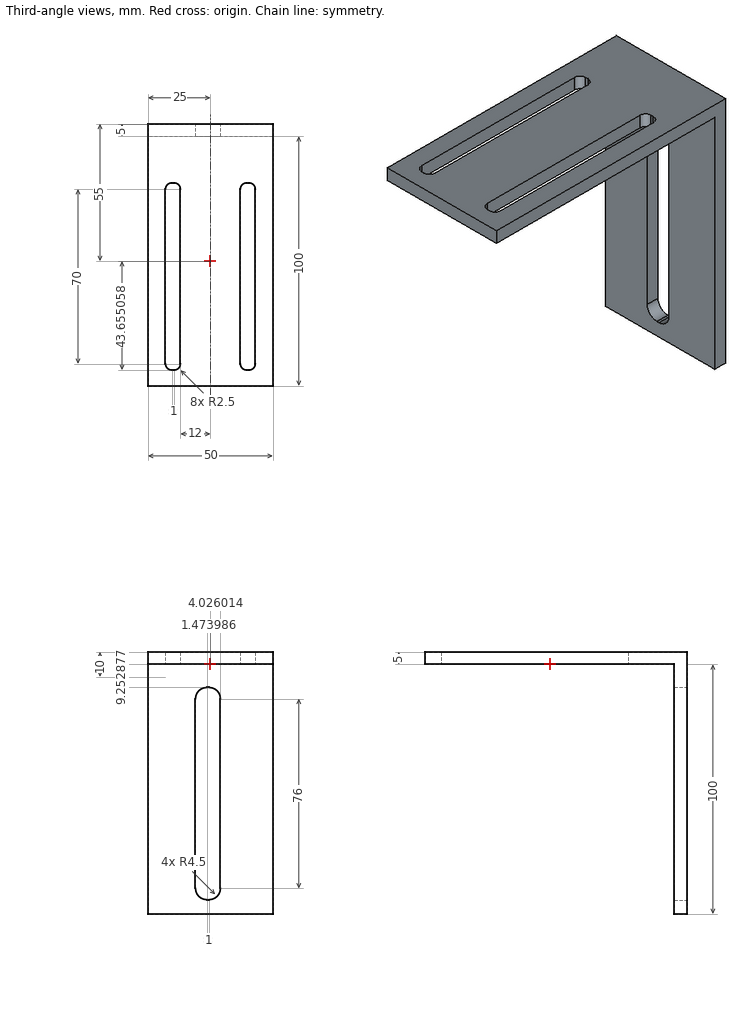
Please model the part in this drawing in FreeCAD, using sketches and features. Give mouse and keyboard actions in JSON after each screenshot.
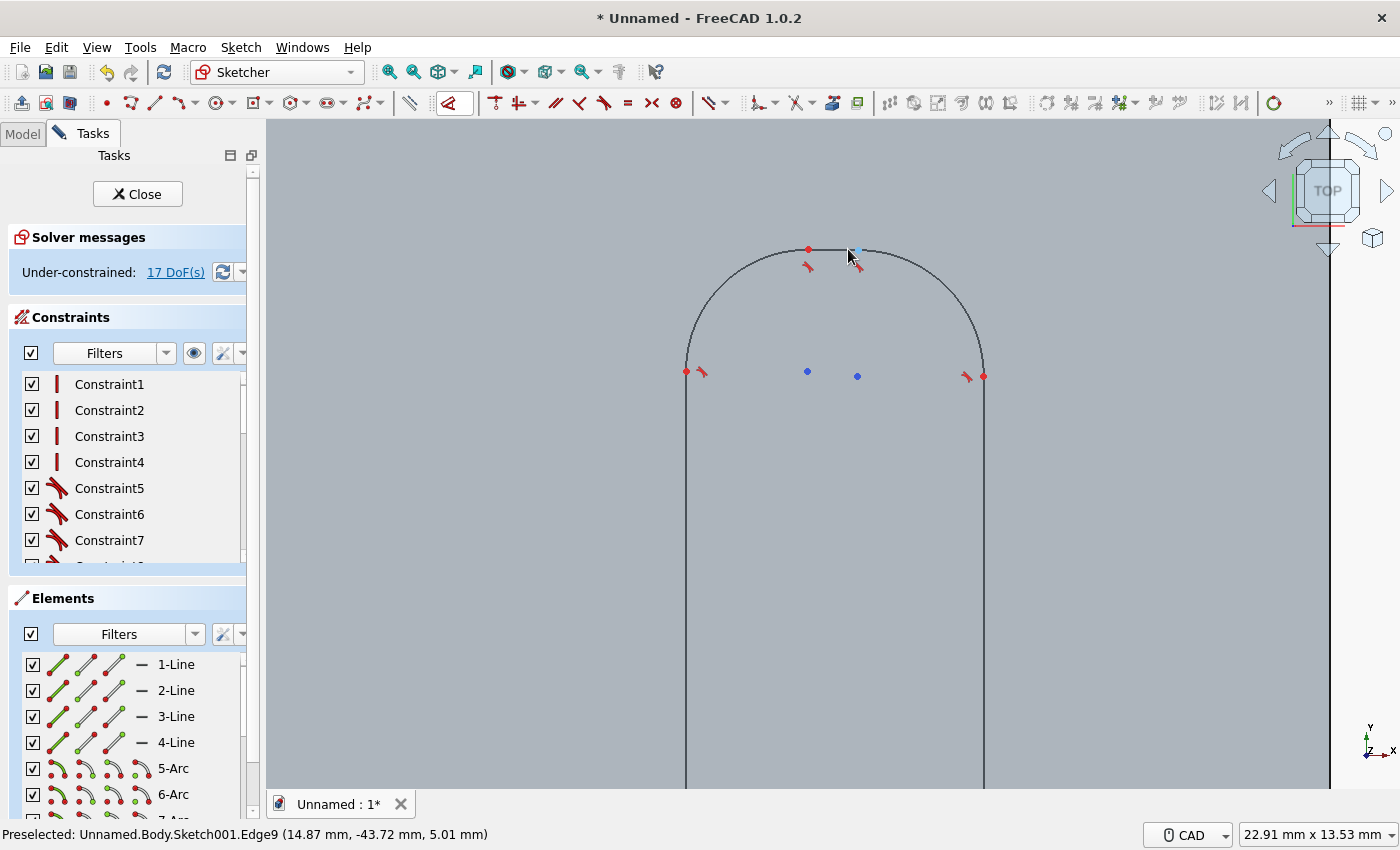
{"action": "left_click", "coordinate": [843, 250]}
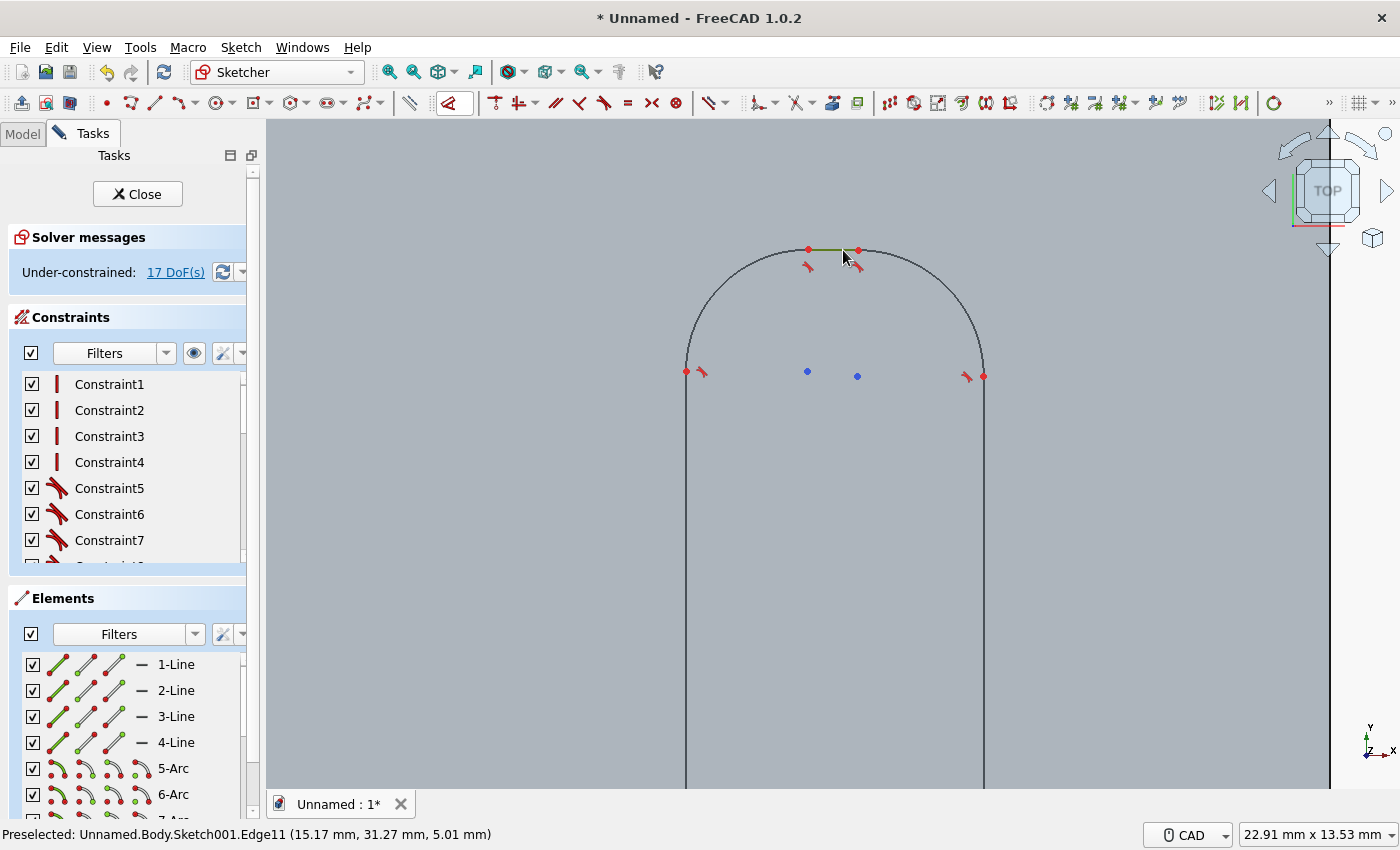
{"action": "key", "text": "h"}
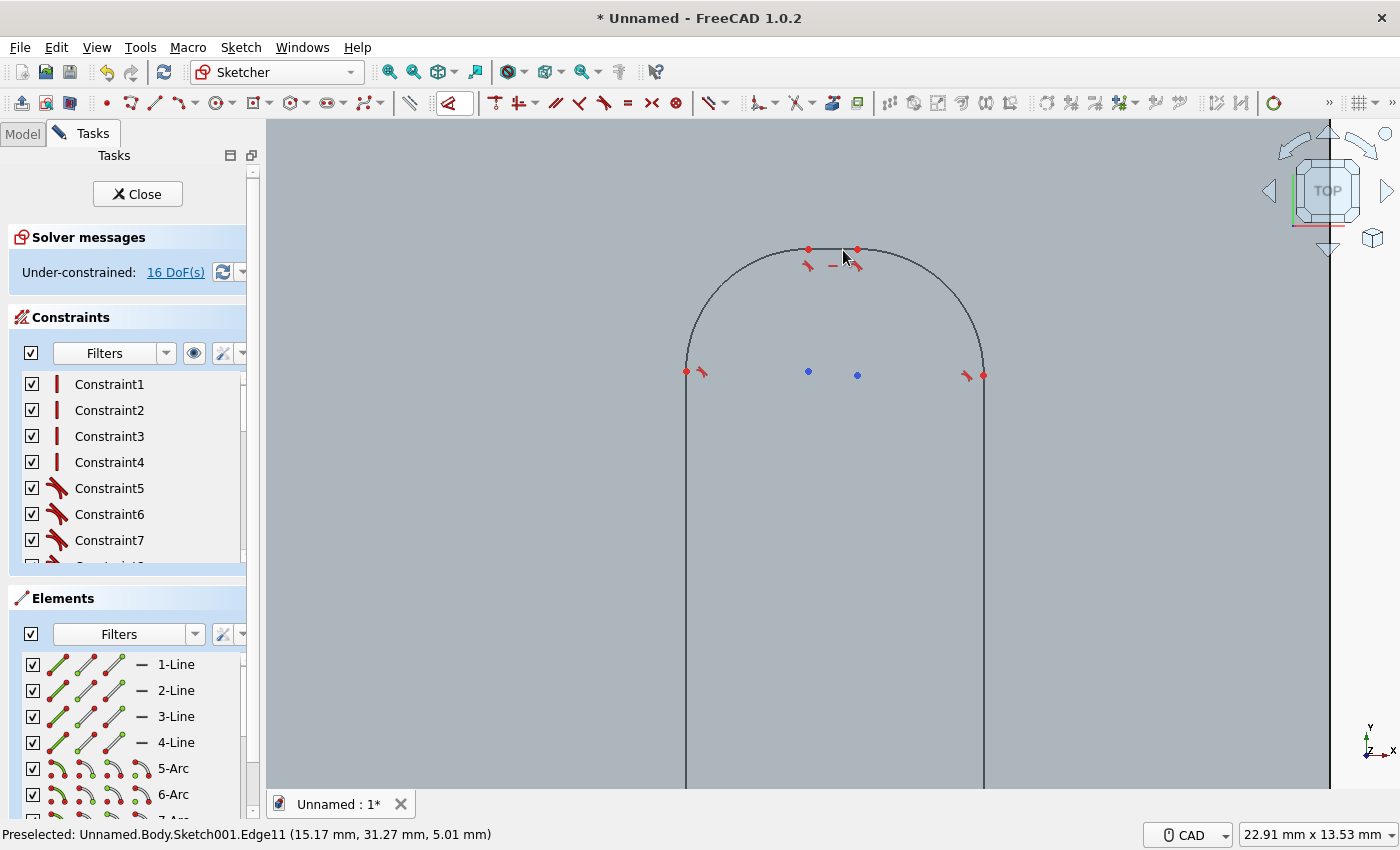
{"action": "scroll", "coordinate": [848, 249], "scroll_direction": "down", "scroll_amount": 11}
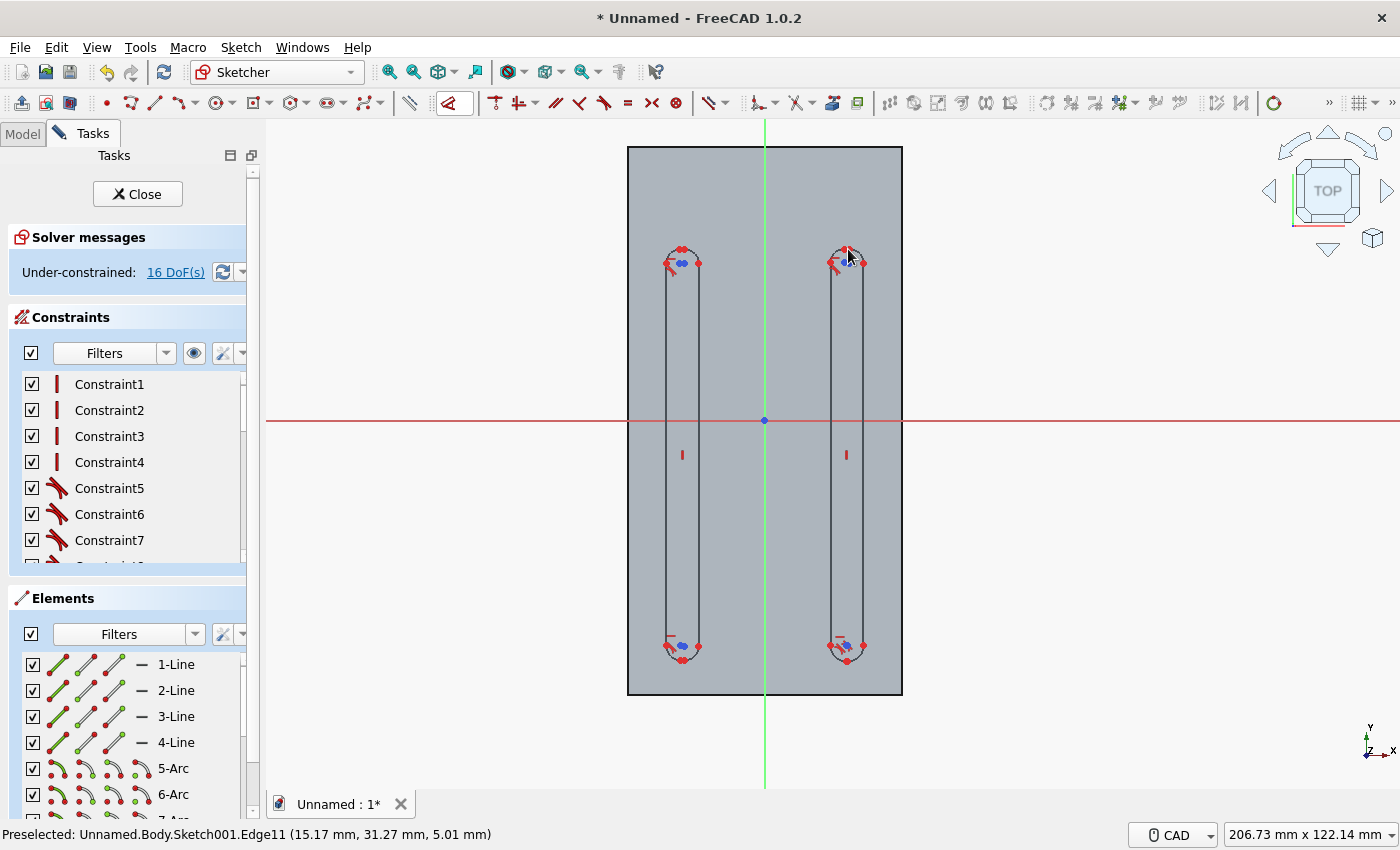
{"action": "scroll", "coordinate": [691, 659], "scroll_direction": "up", "scroll_amount": 4}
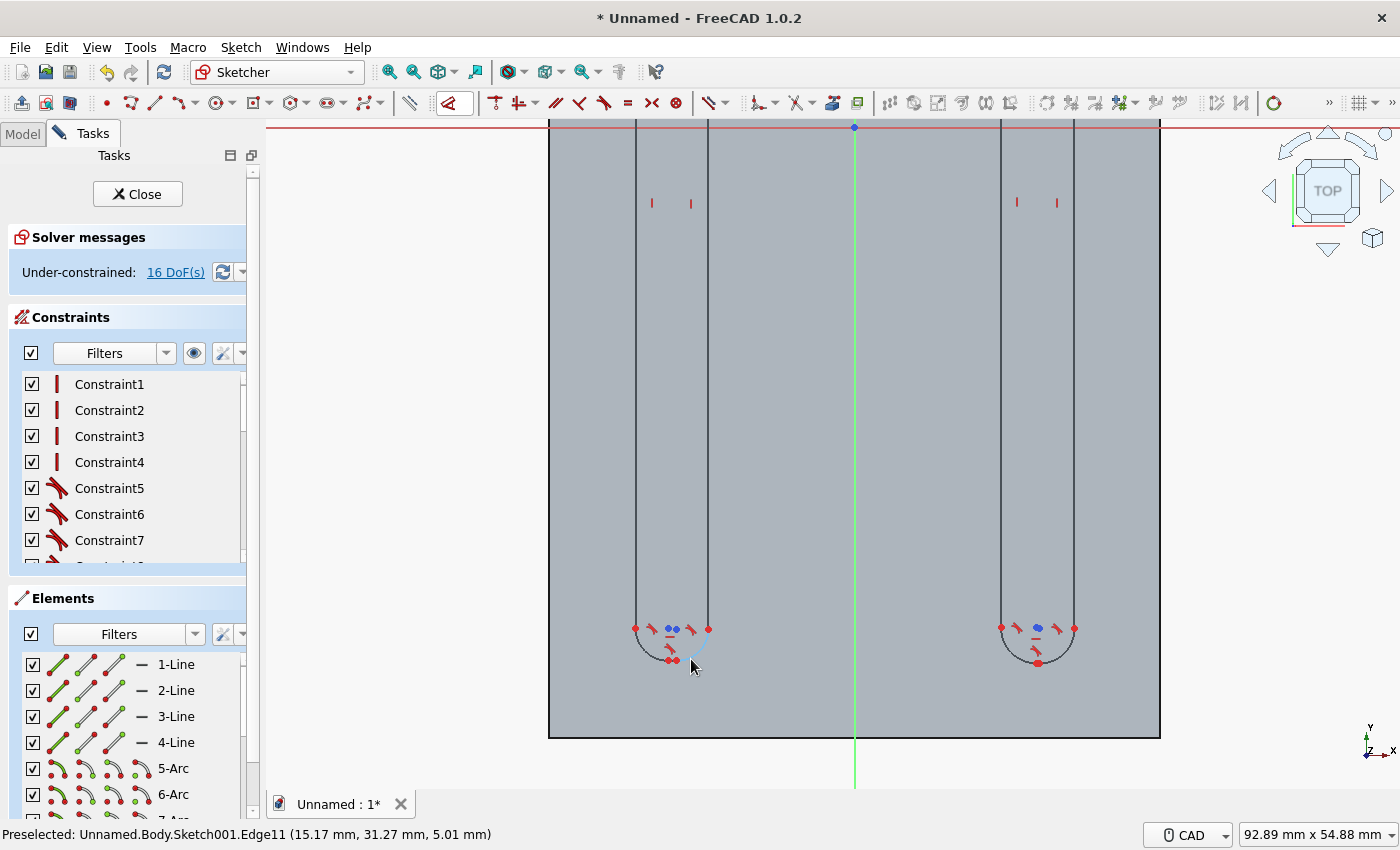
{"action": "left_click", "coordinate": [691, 657]}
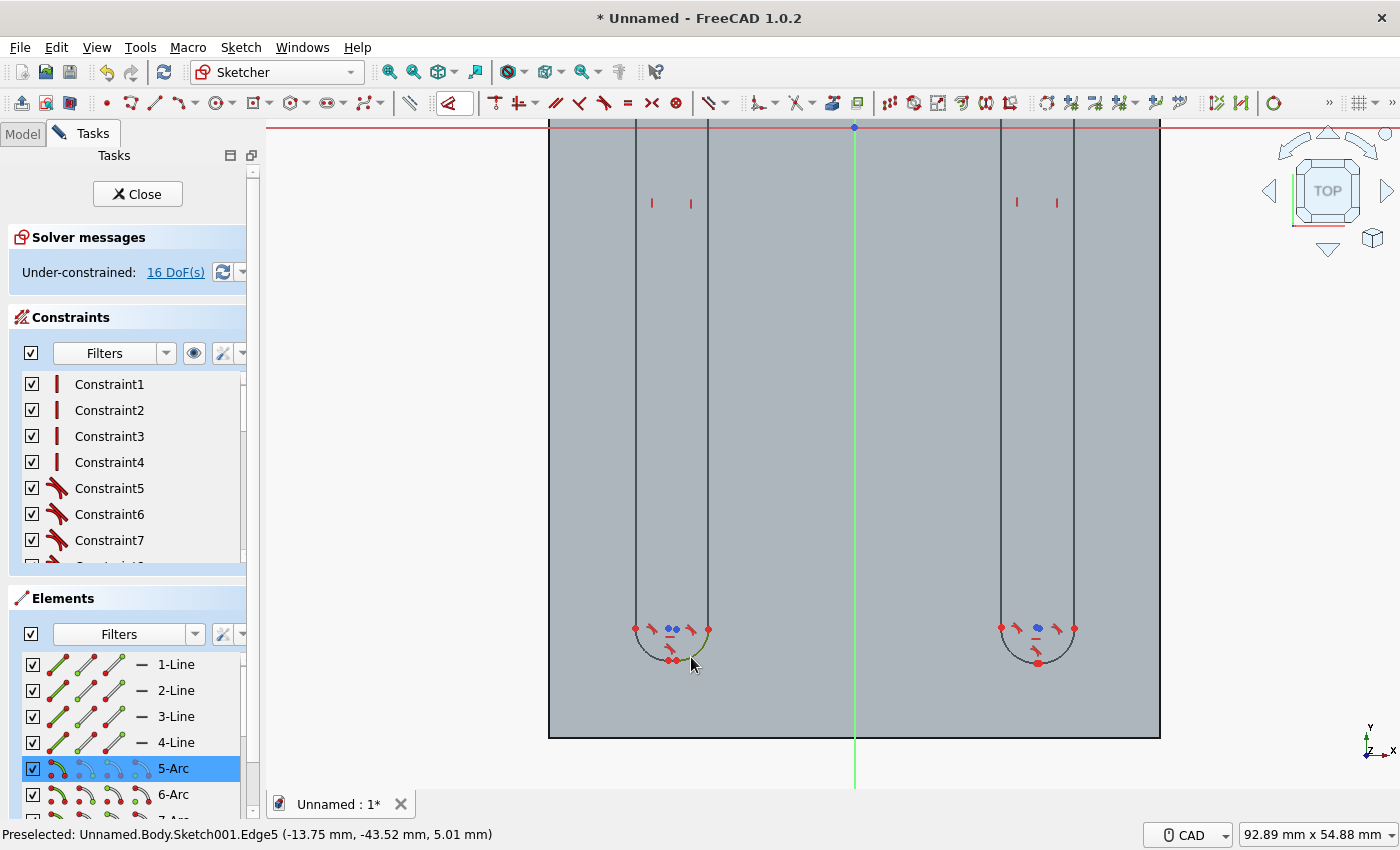
{"action": "scroll", "coordinate": [691, 659], "scroll_direction": "down", "scroll_amount": 4}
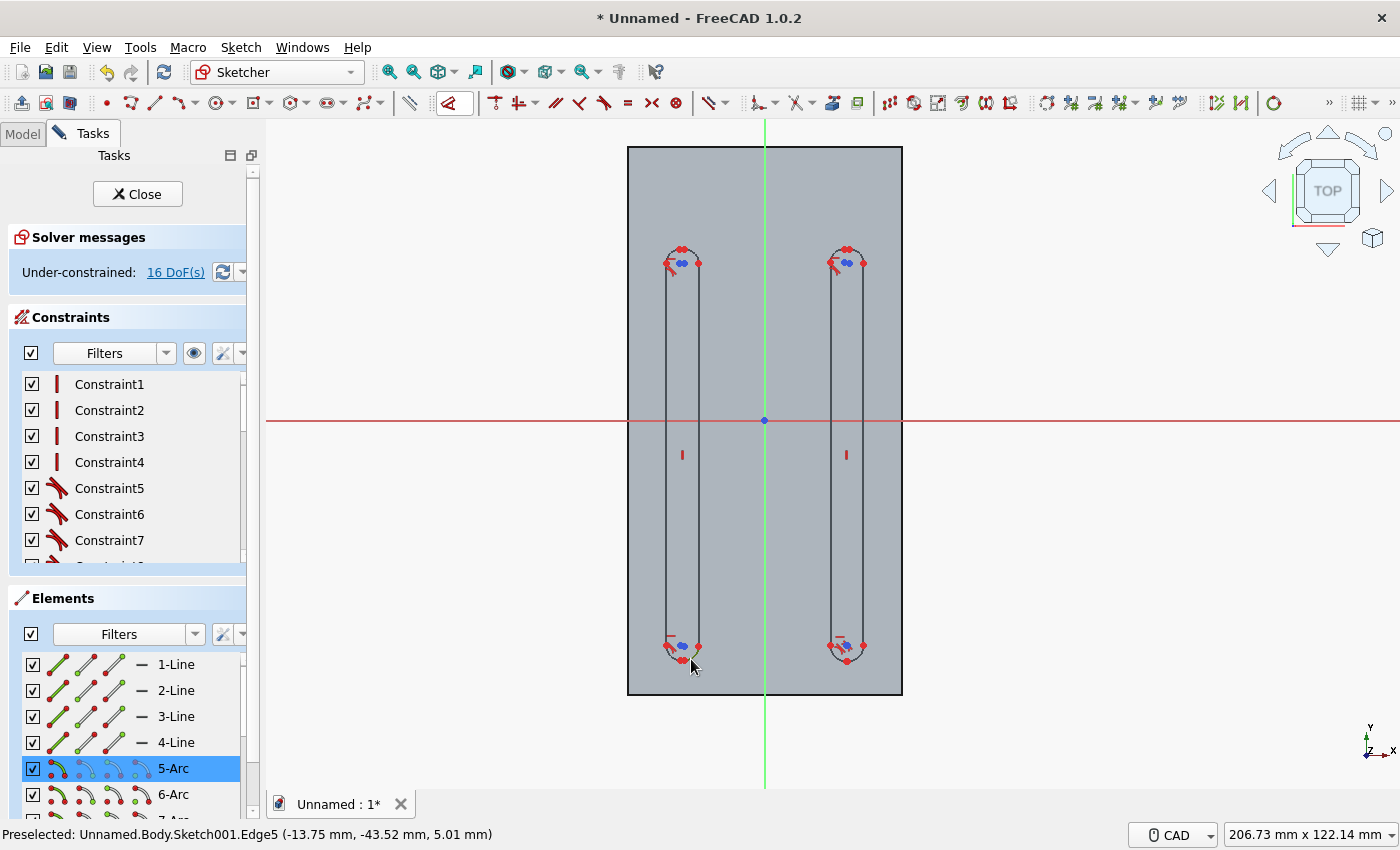
{"action": "scroll", "coordinate": [697, 257], "scroll_direction": "up", "scroll_amount": 4}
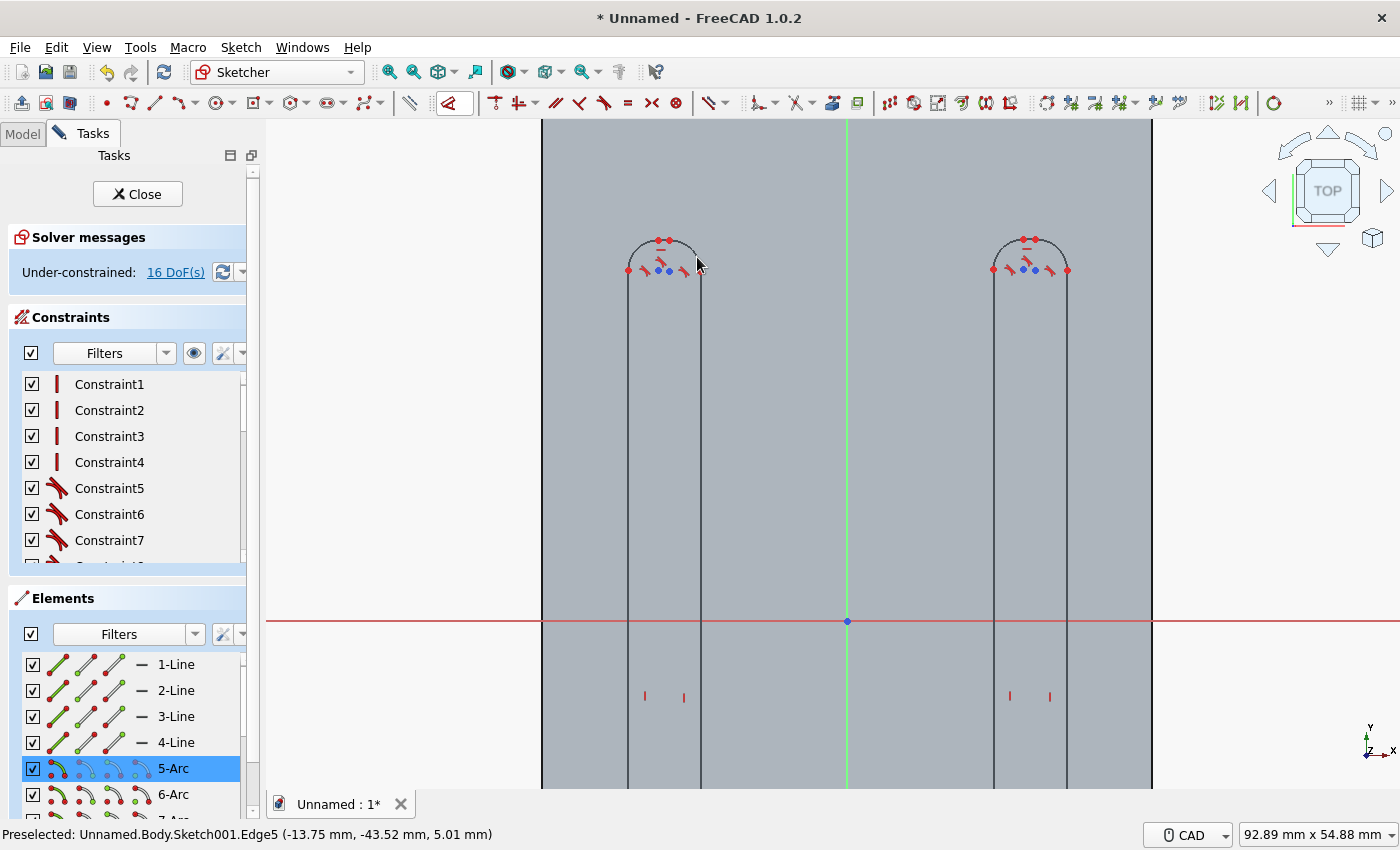
{"action": "left_click", "coordinate": [698, 257]}